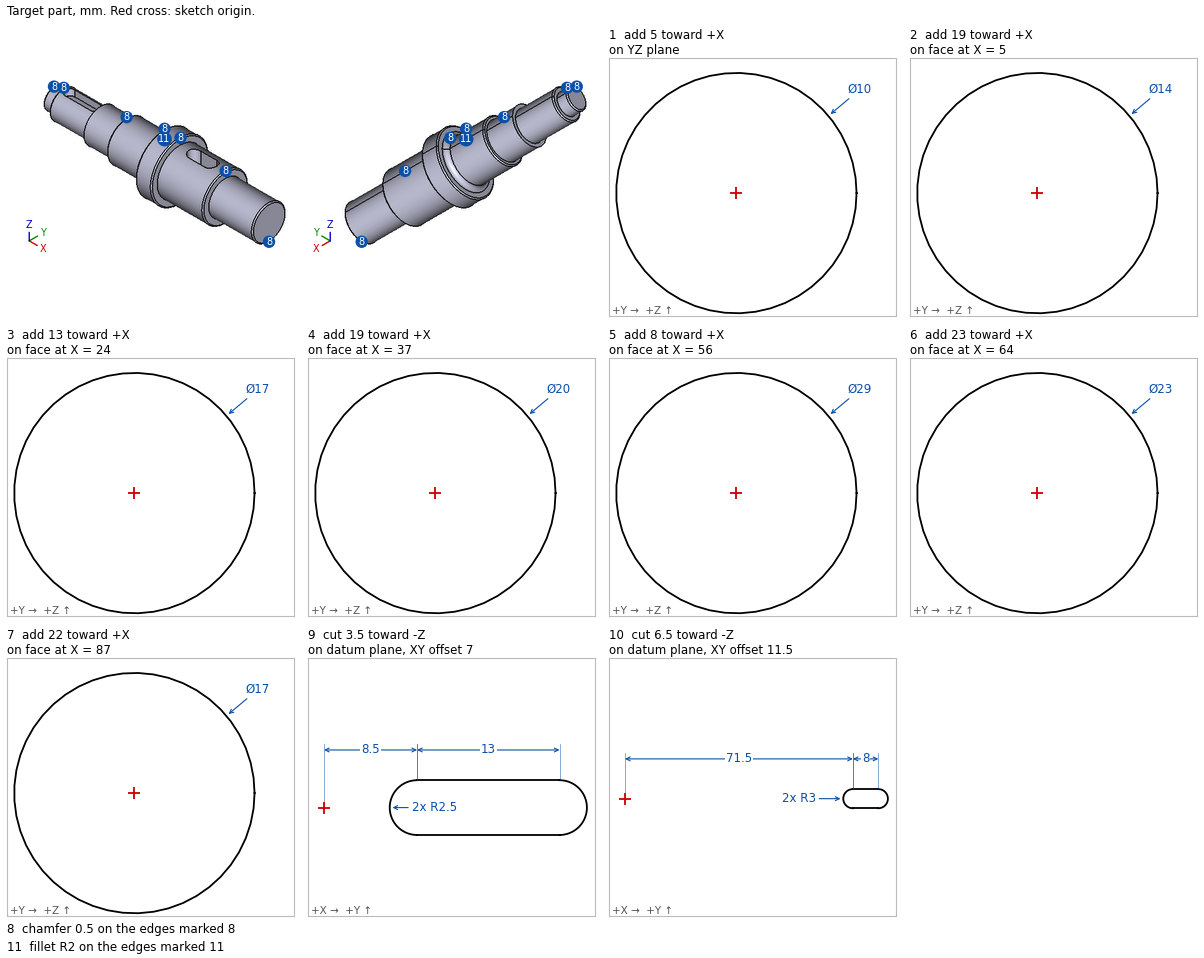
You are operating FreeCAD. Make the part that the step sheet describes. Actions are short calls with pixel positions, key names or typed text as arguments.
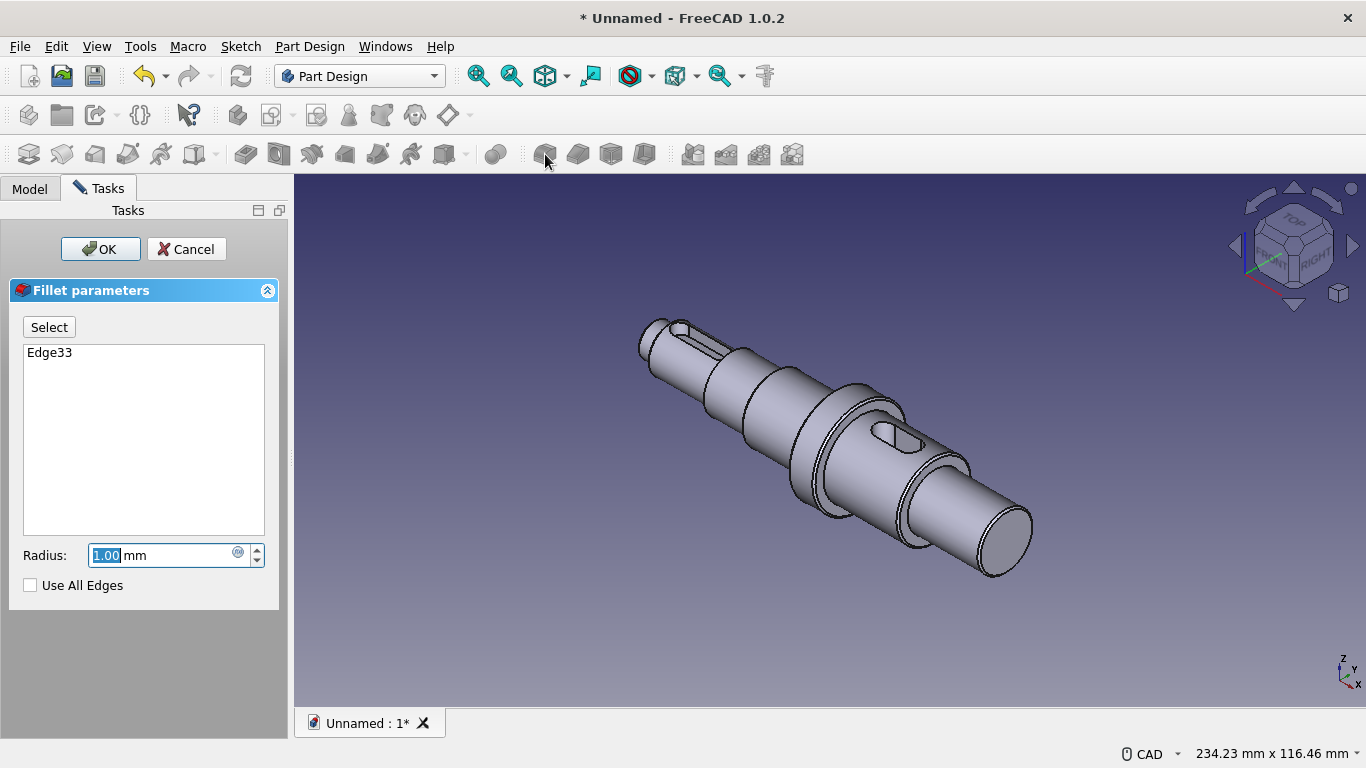
text(2)
key(Tab)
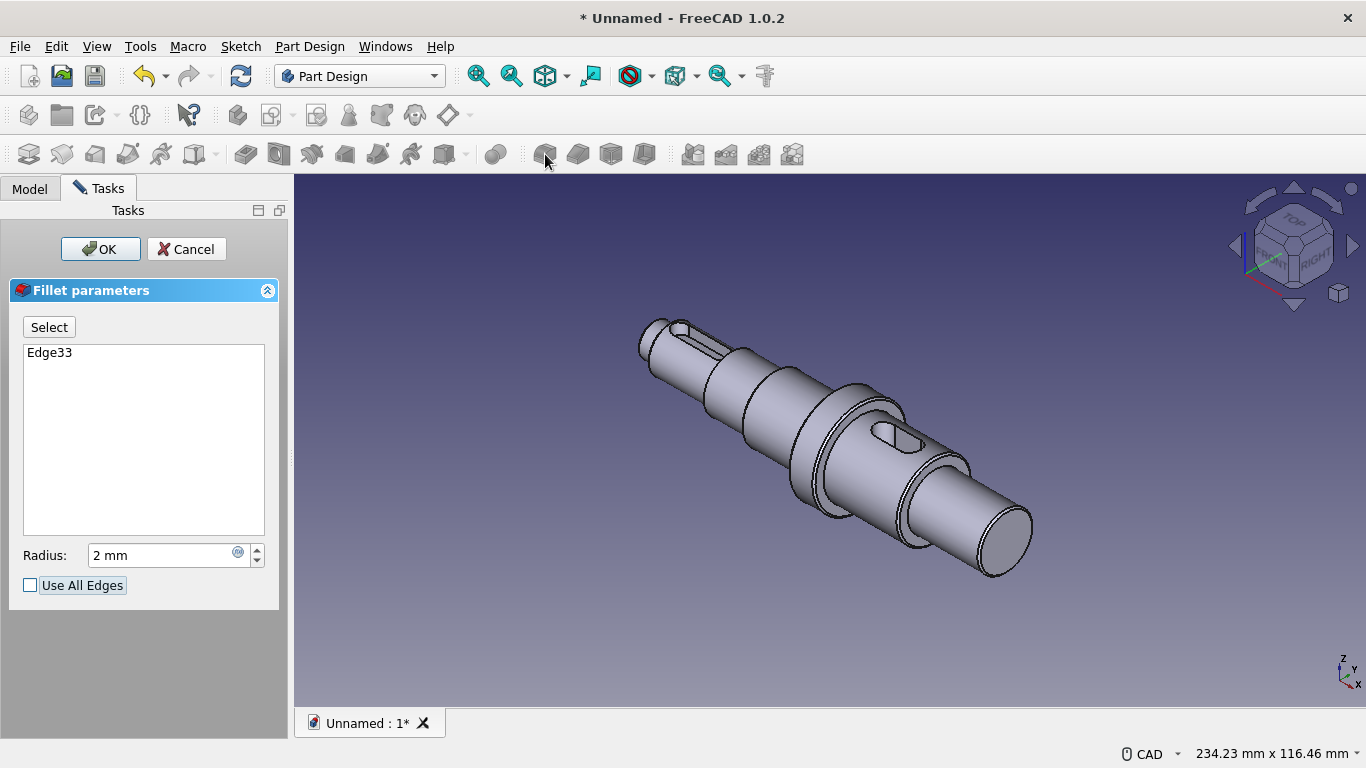
click(101, 249)